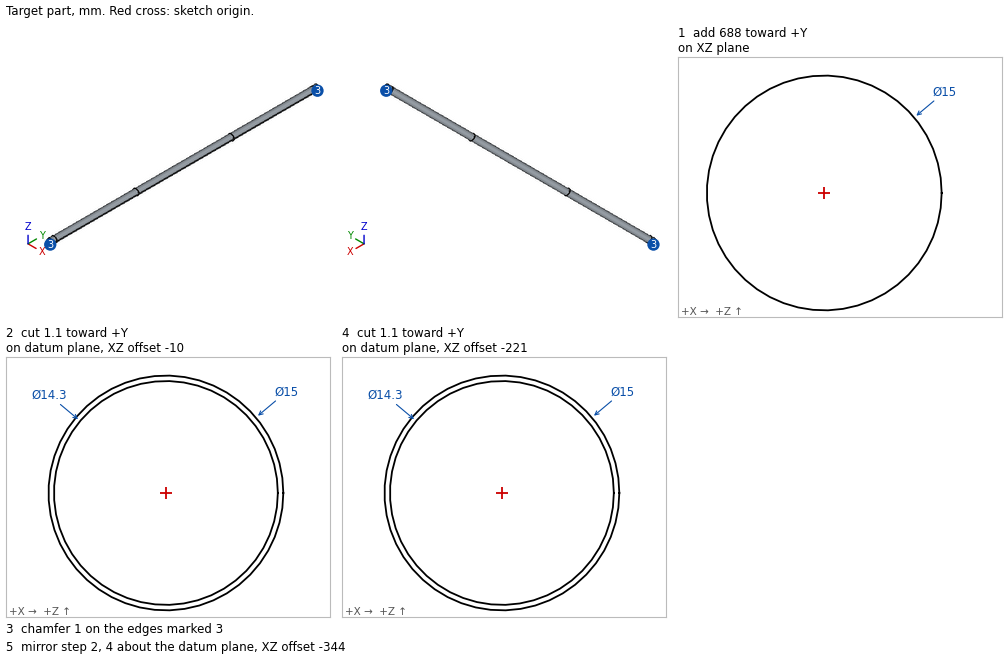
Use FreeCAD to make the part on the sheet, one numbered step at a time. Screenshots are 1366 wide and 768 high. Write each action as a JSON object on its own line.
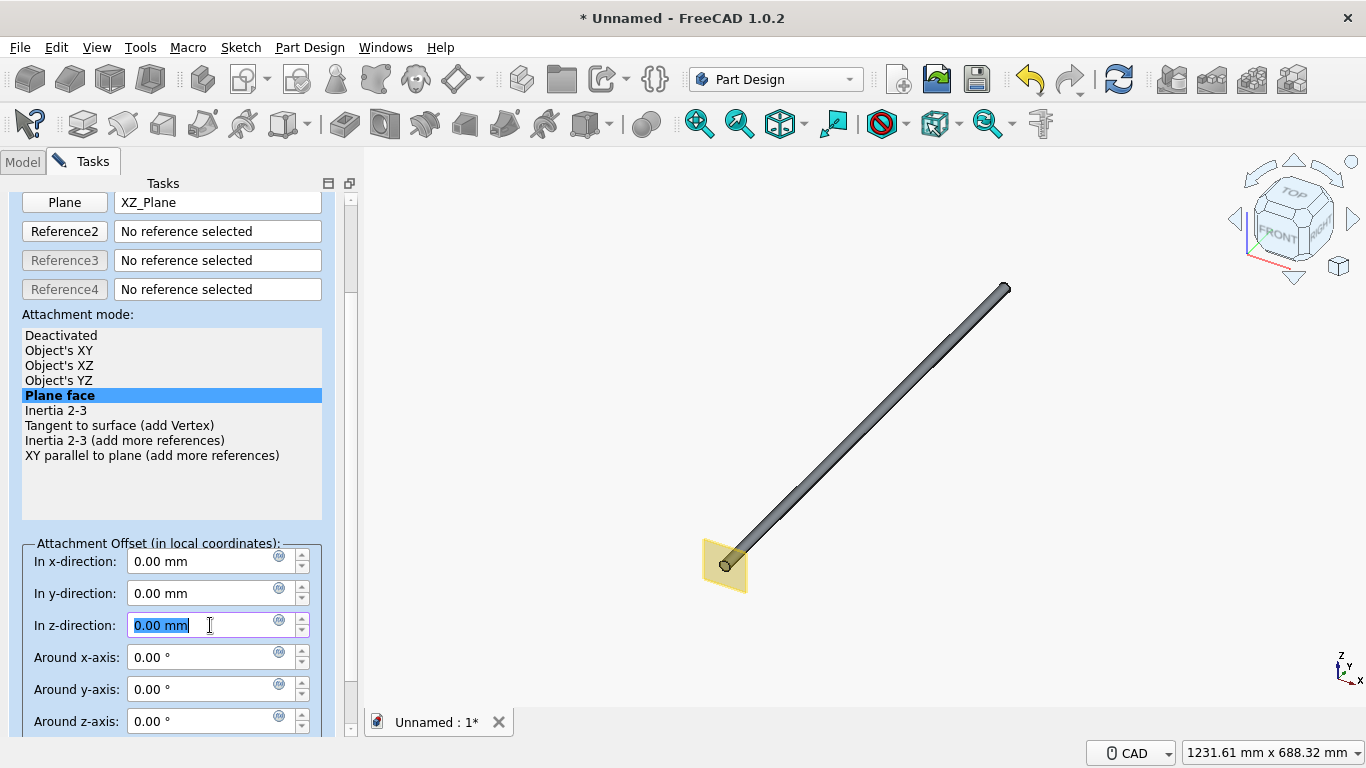
{"action": "type", "text": "-10"}
{"action": "key", "text": "Tab"}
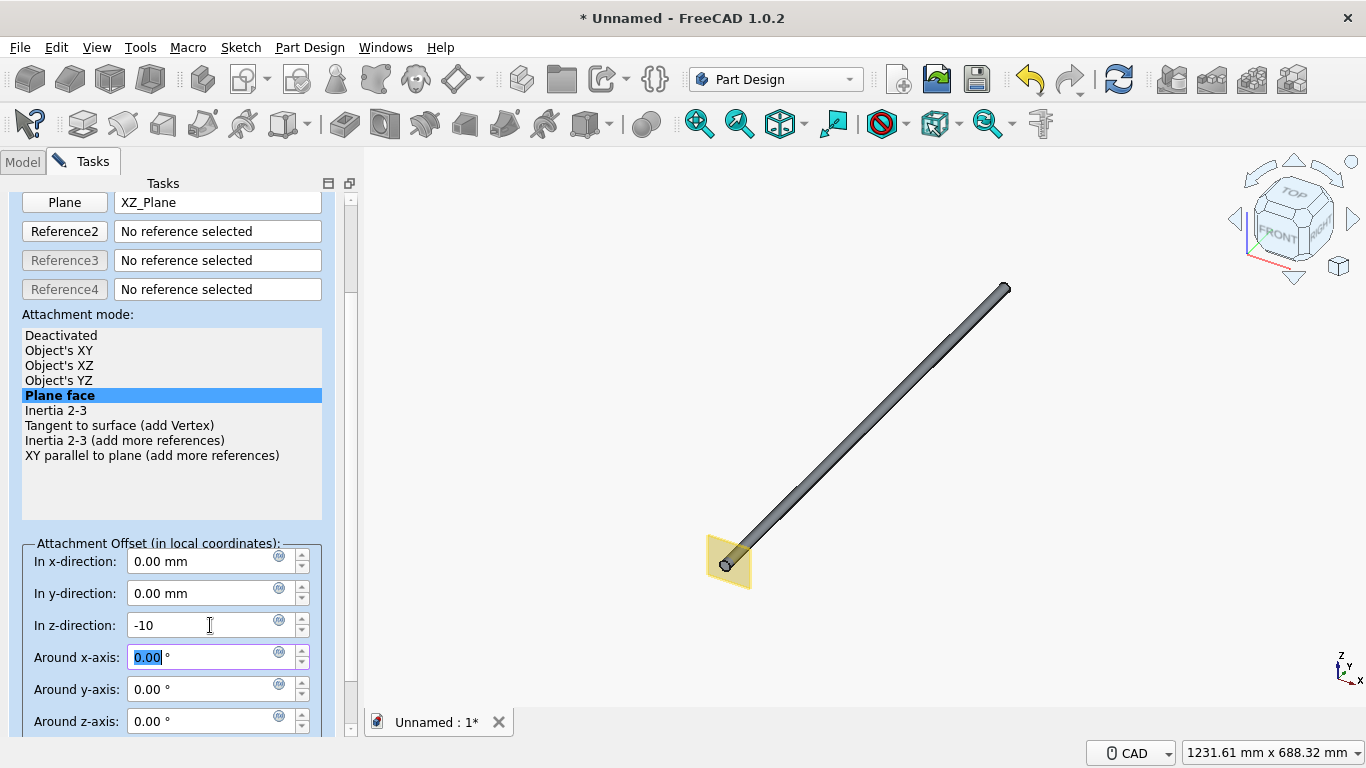
{"action": "scroll", "coordinate": [351, 464], "scroll_direction": "up", "scroll_amount": 3}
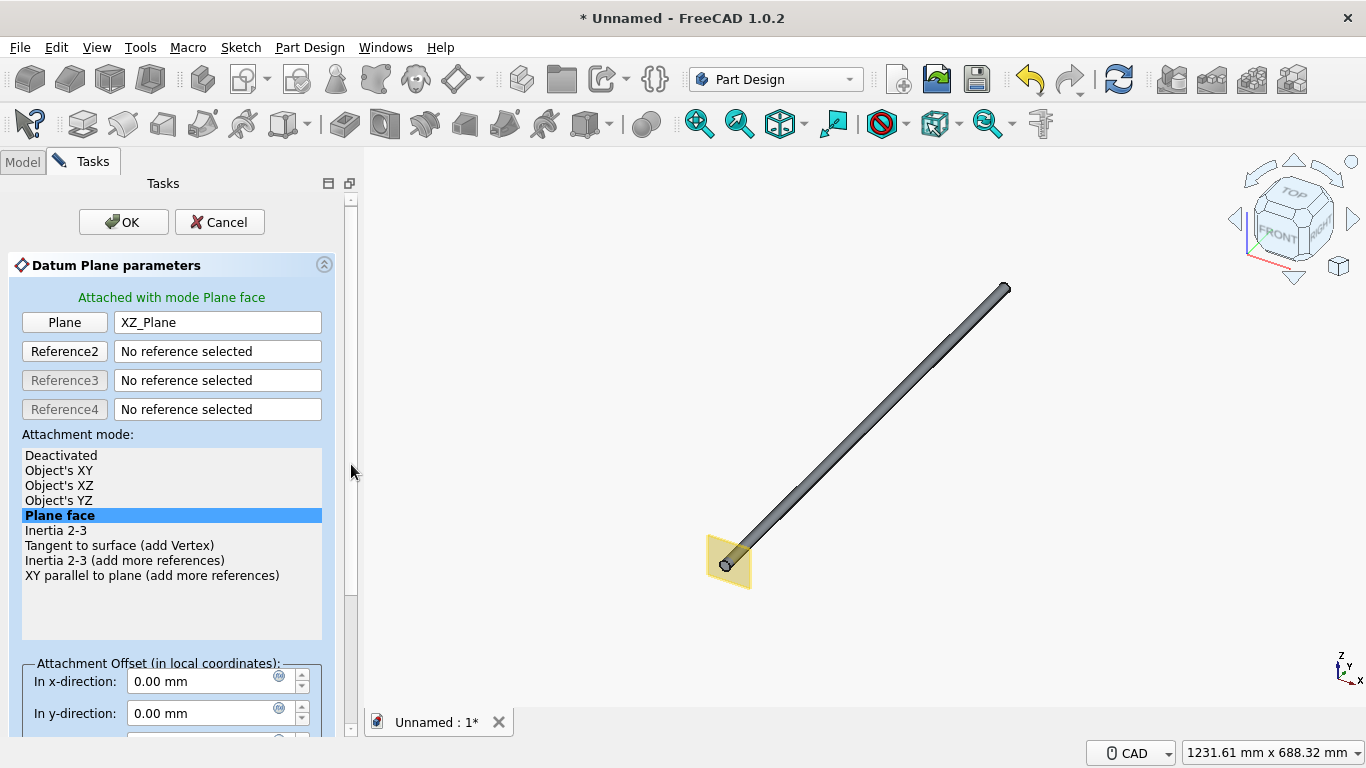
{"action": "left_click", "coordinate": [124, 222]}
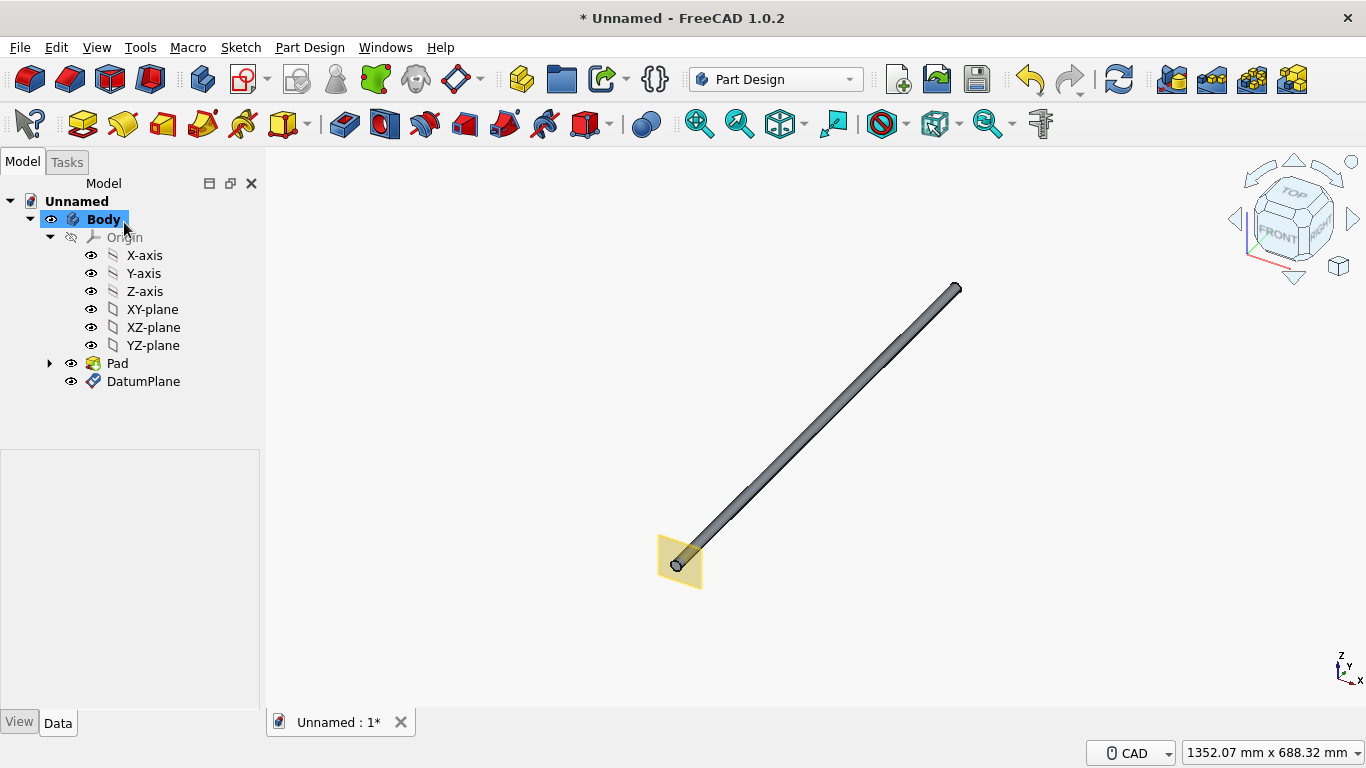
{"action": "left_click", "coordinate": [116, 381]}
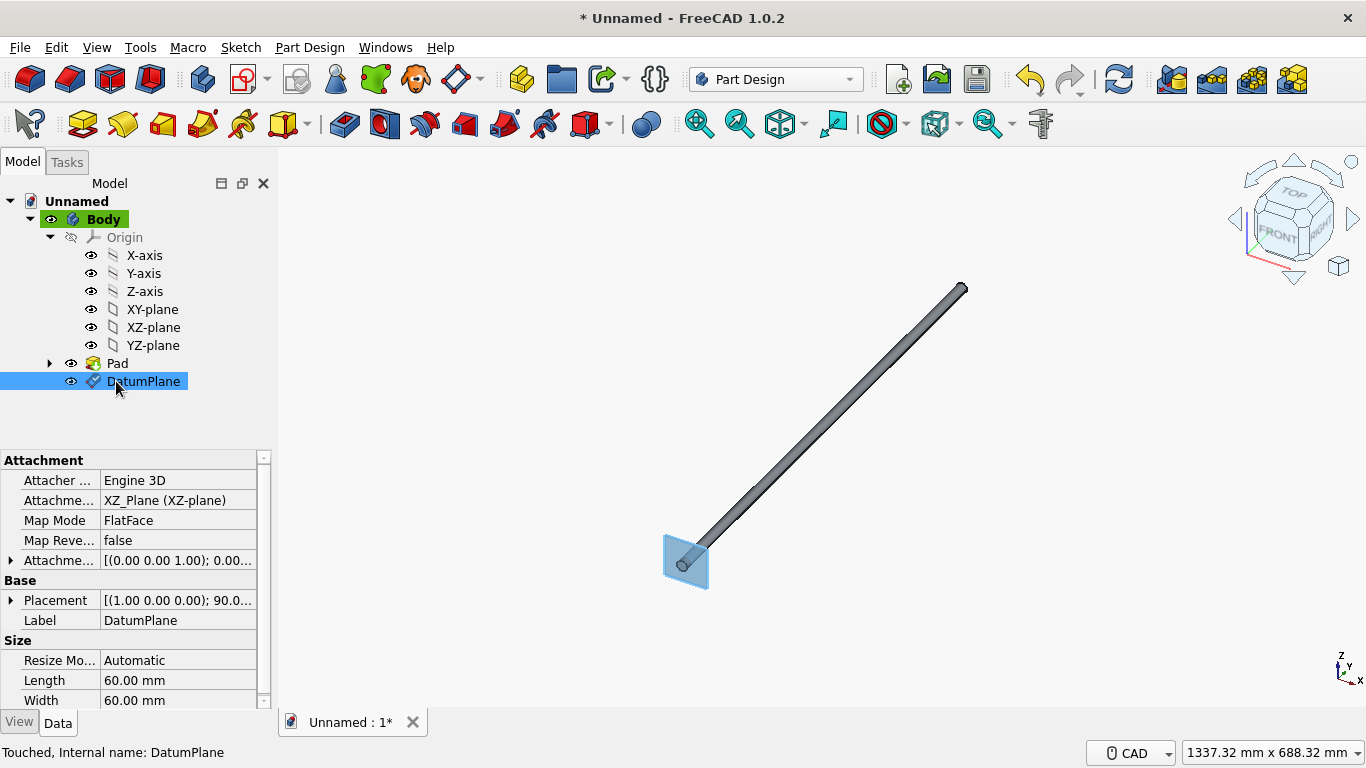
{"action": "left_click", "coordinate": [244, 80]}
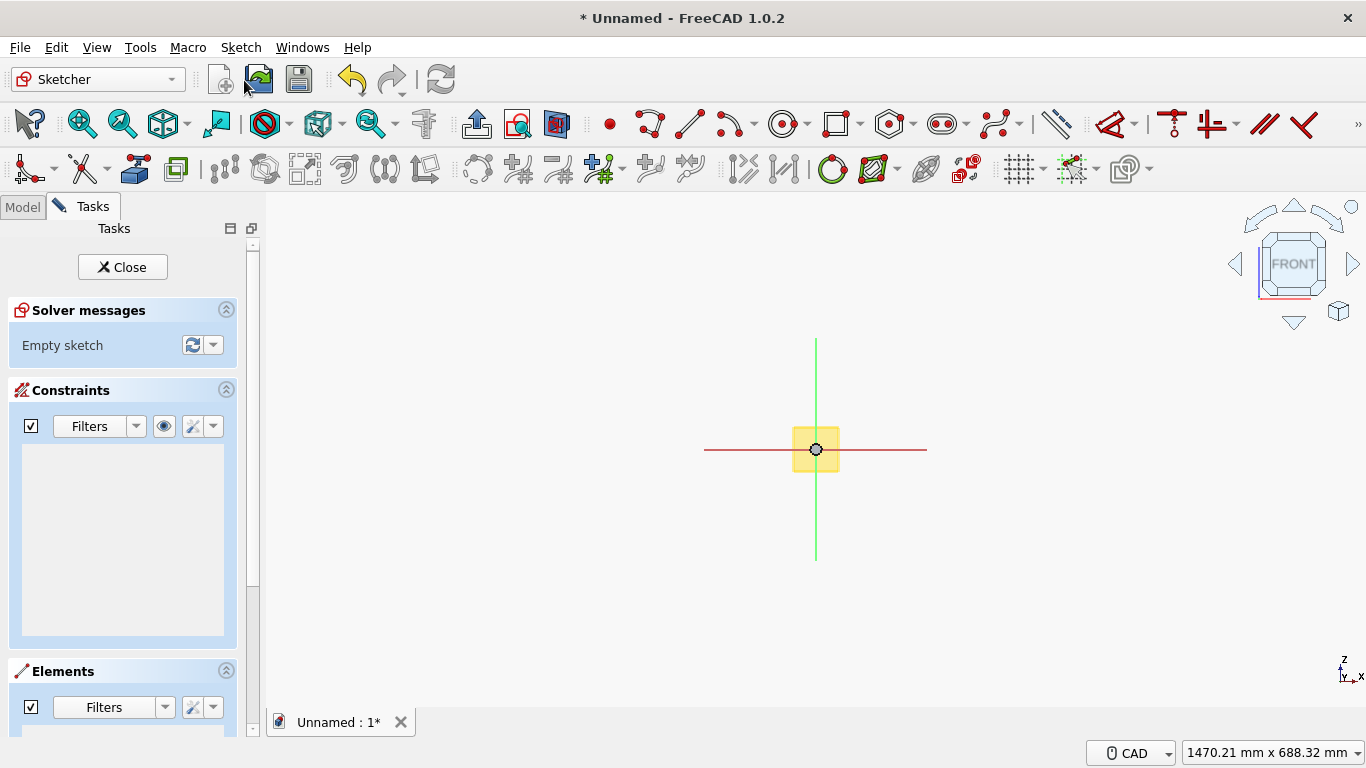
{"action": "left_click", "coordinate": [558, 124]}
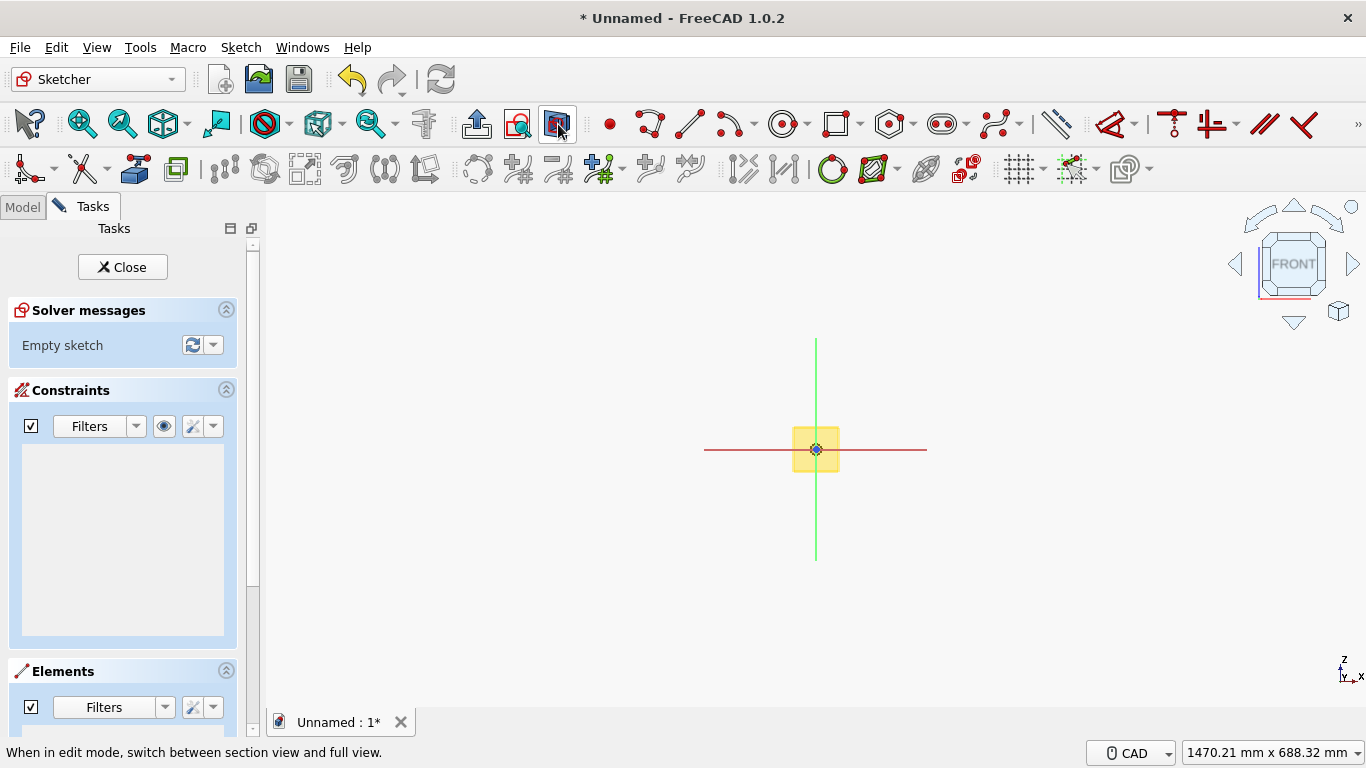
{"action": "scroll", "coordinate": [820, 450], "scroll_direction": "up", "scroll_amount": 15}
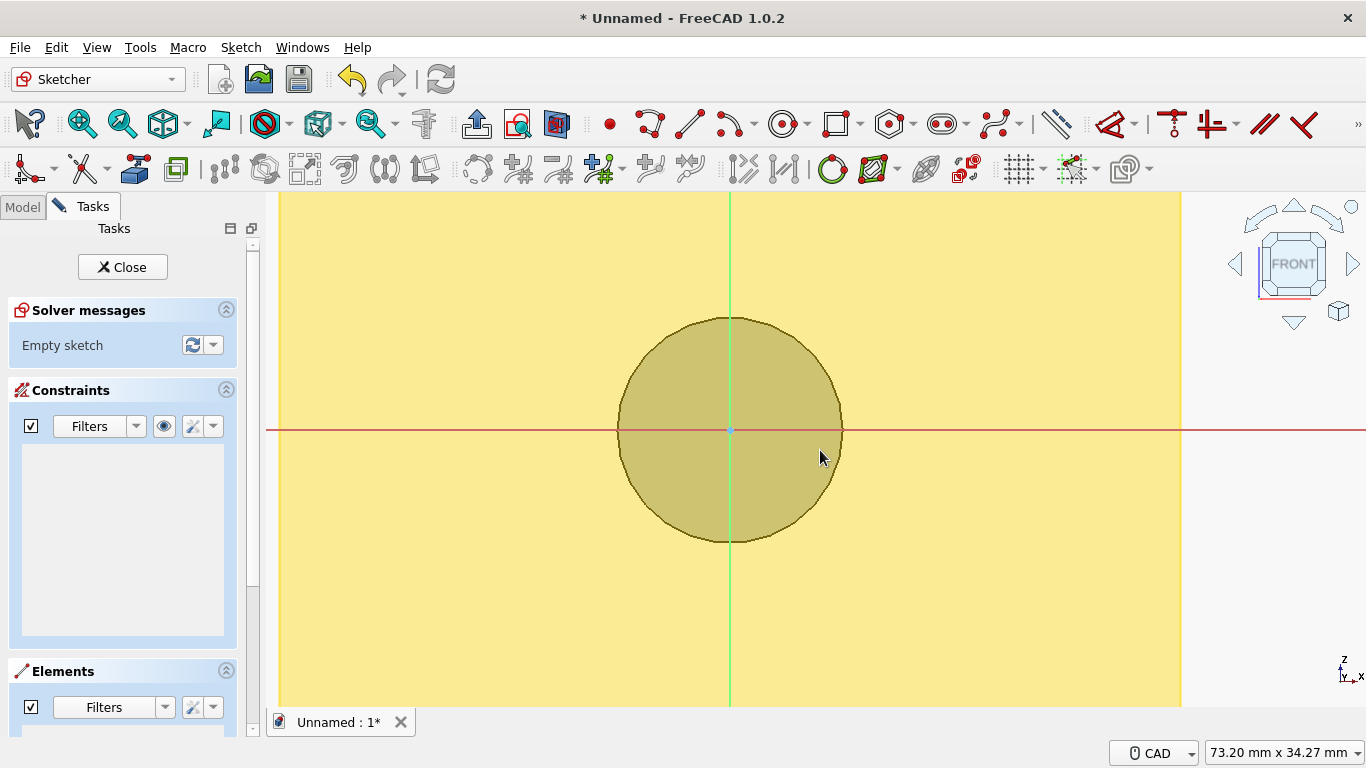
{"action": "scroll", "coordinate": [695, 391], "scroll_direction": "up", "scroll_amount": 2}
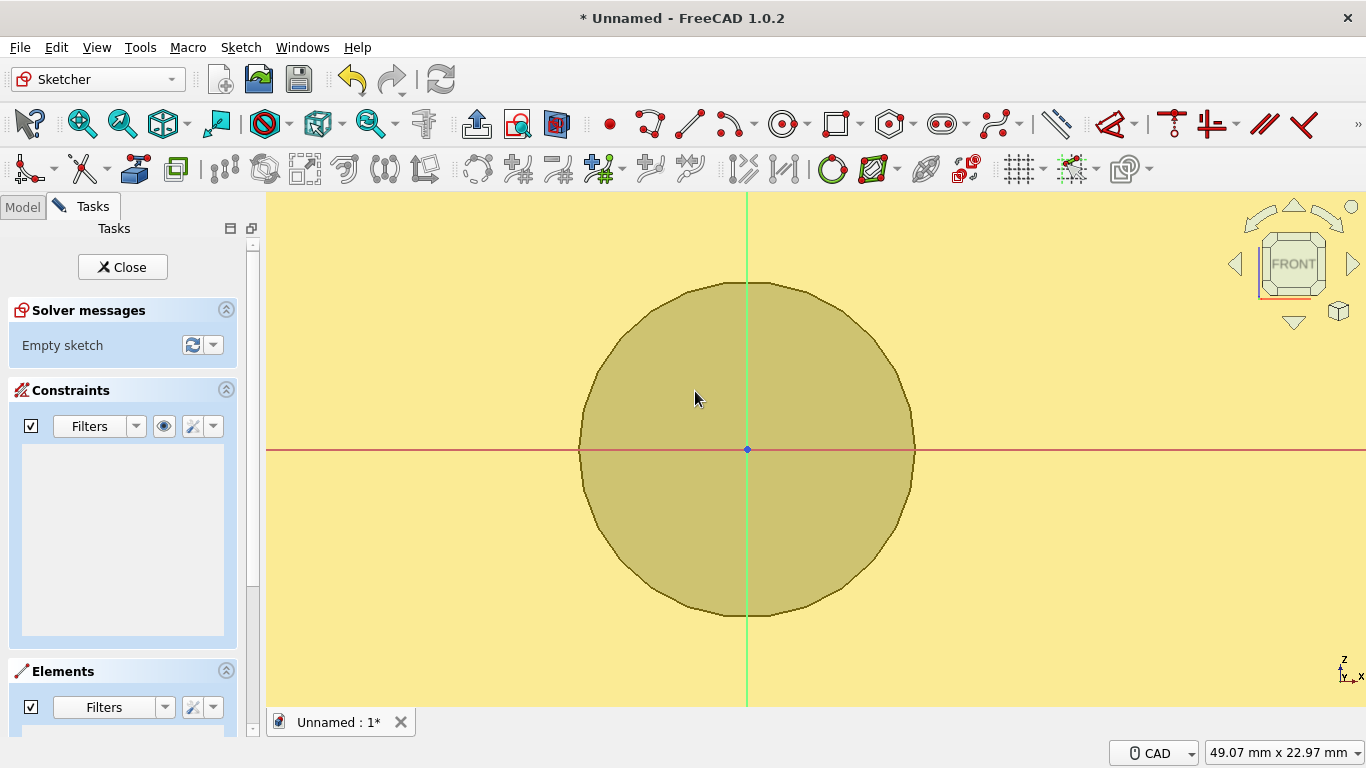
{"action": "left_click", "coordinate": [784, 124]}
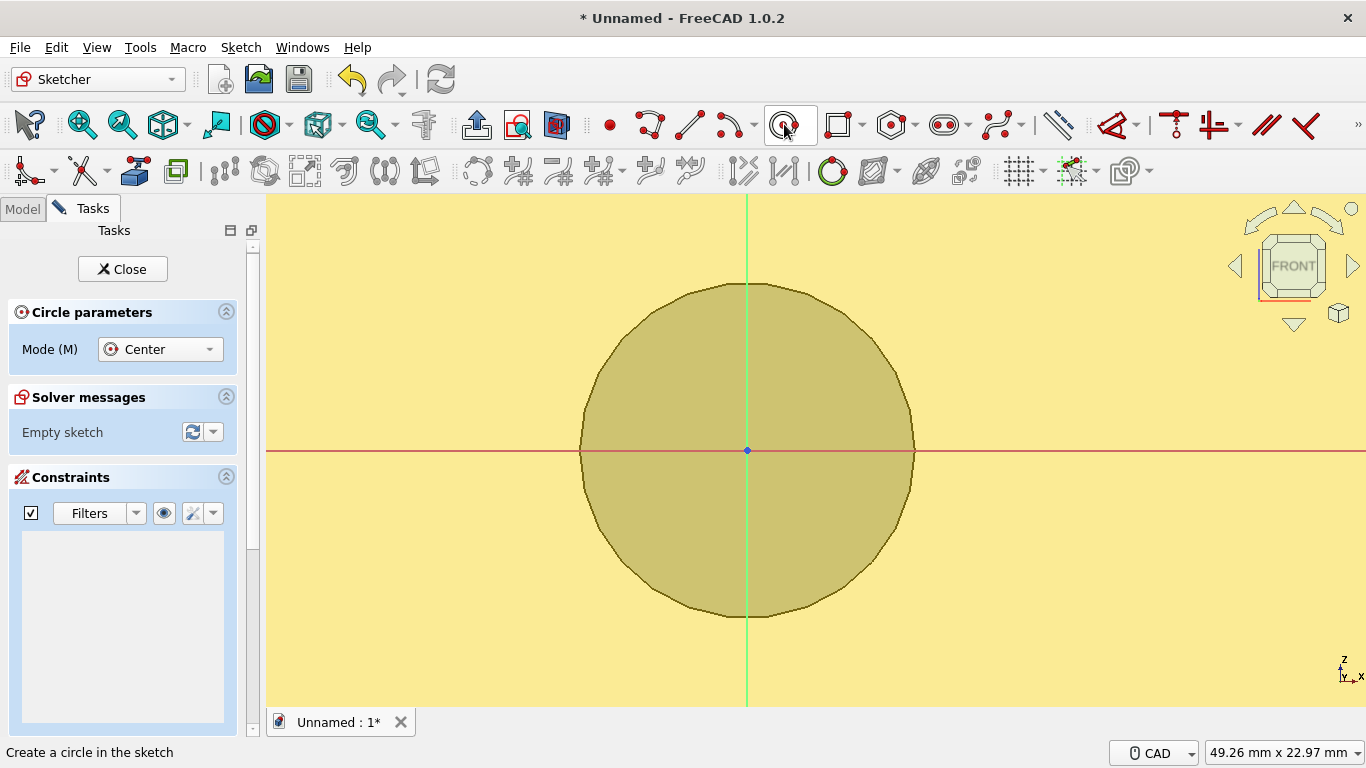
{"action": "left_click", "coordinate": [747, 451]}
{"action": "mouse_move", "coordinate": [866, 332]}